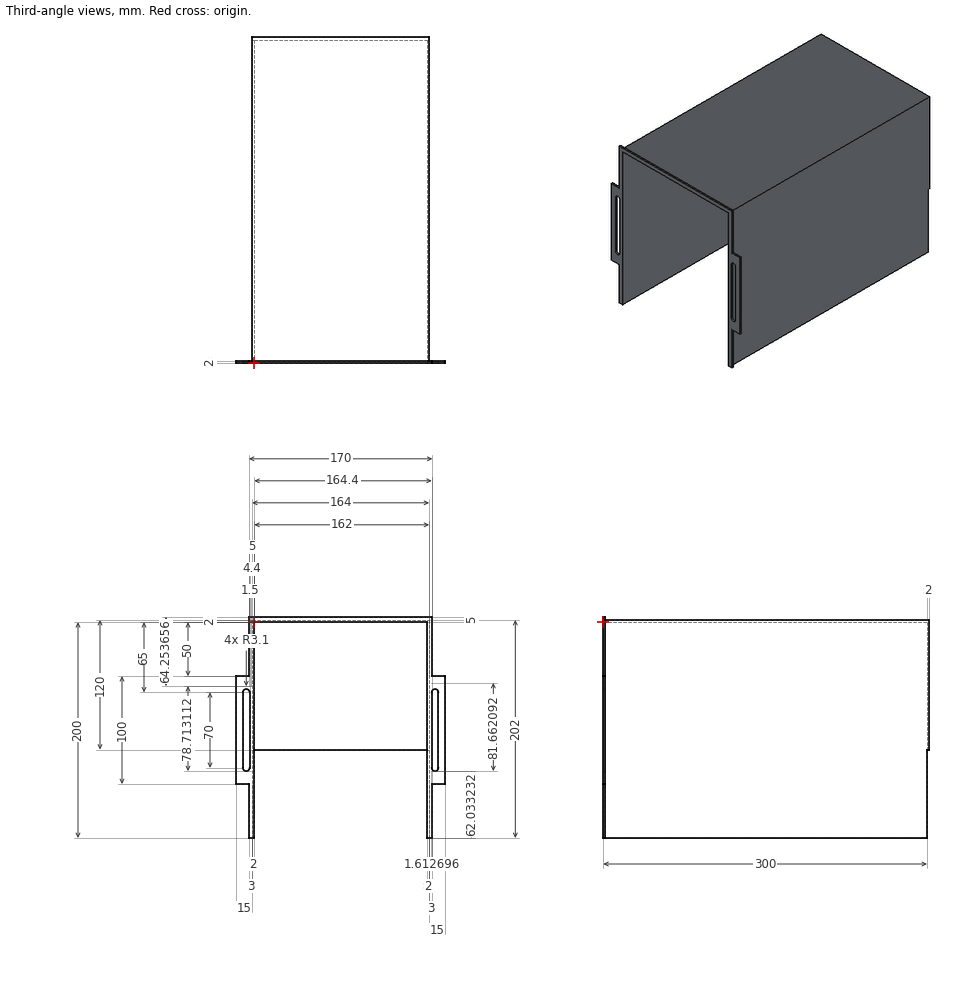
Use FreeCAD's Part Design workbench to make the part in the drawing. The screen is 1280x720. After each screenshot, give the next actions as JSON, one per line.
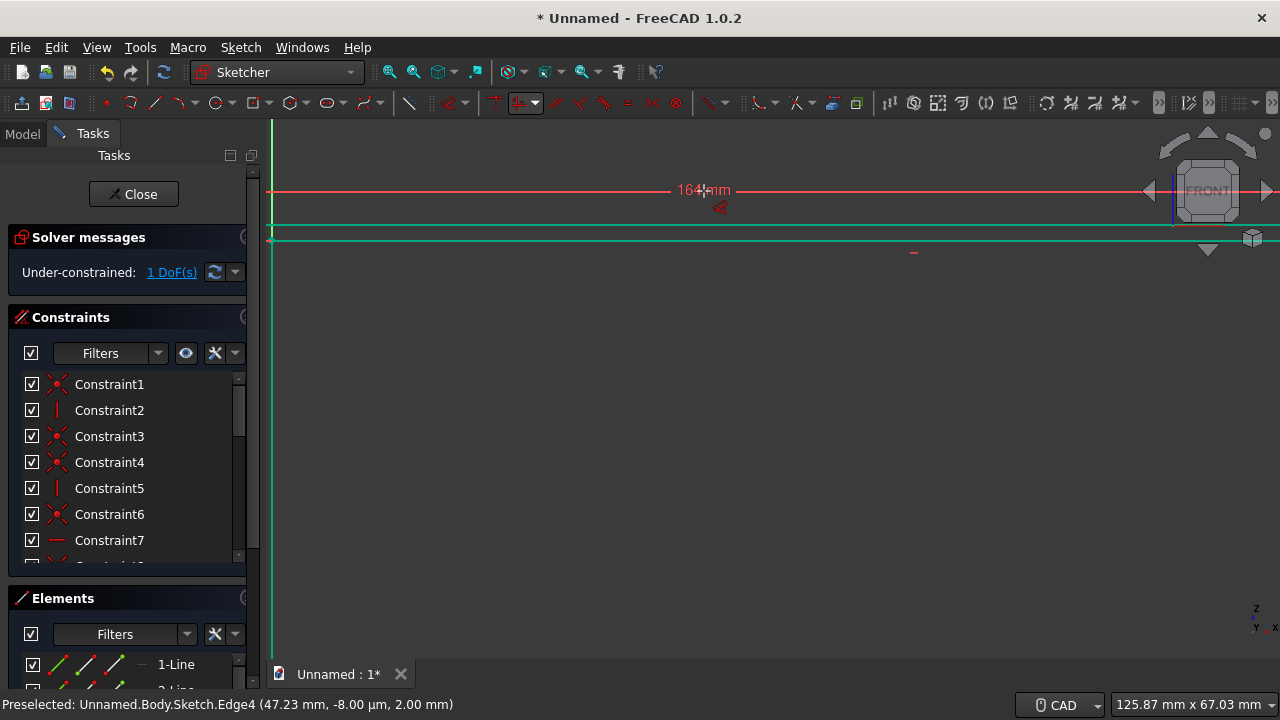
{"action": "scroll", "coordinate": [651, 225], "scroll_direction": "down", "scroll_amount": 8}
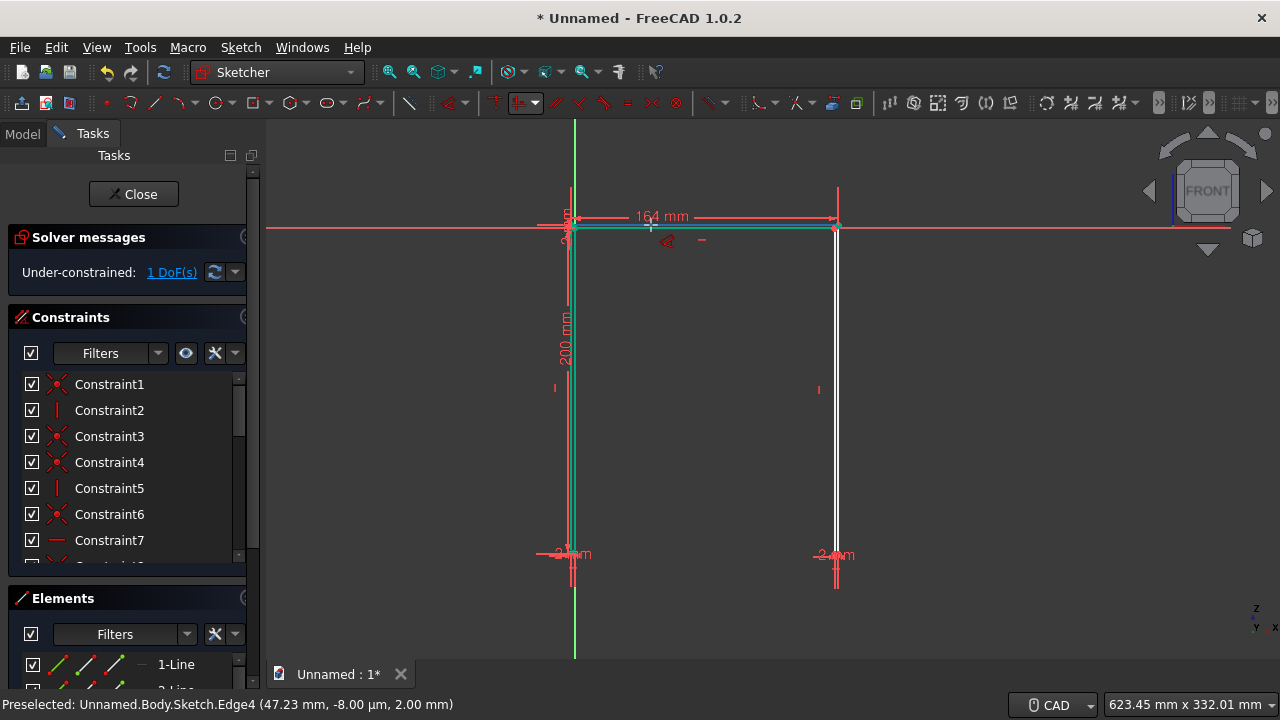
{"action": "scroll", "coordinate": [838, 324], "scroll_direction": "up", "scroll_amount": 8}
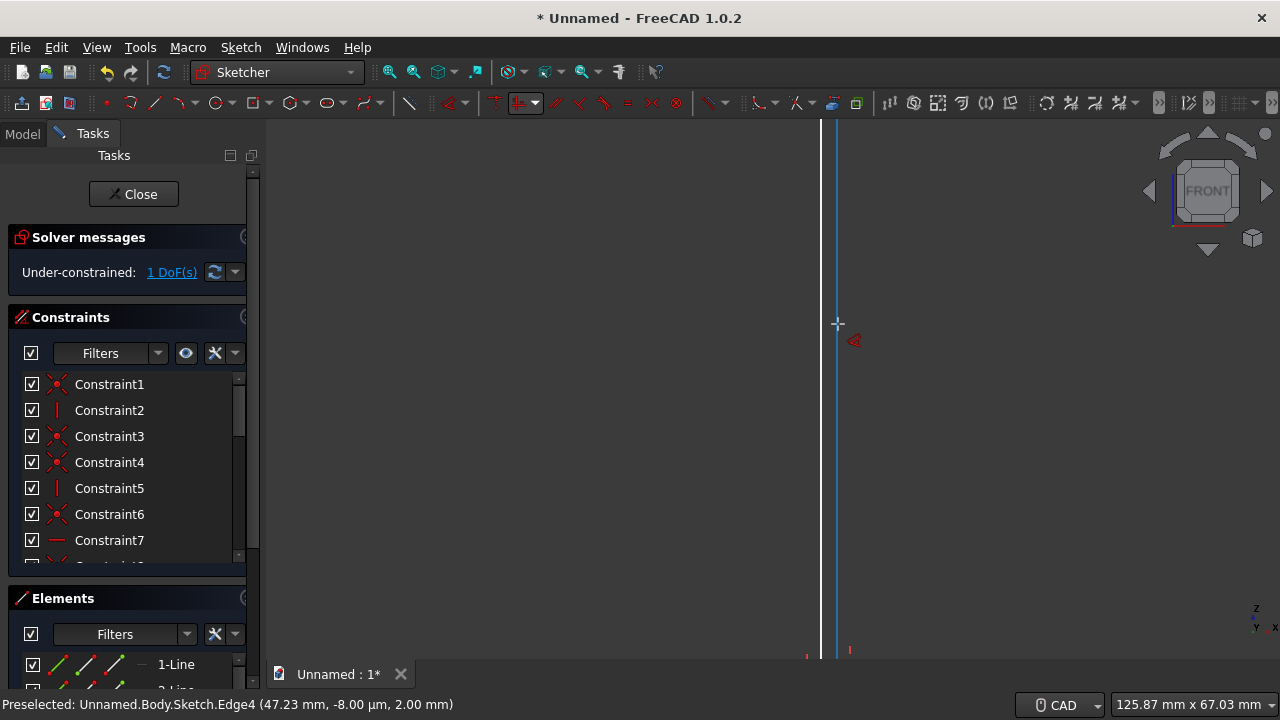
{"action": "left_click", "coordinate": [837, 323]}
{"action": "left_click", "coordinate": [871, 389]}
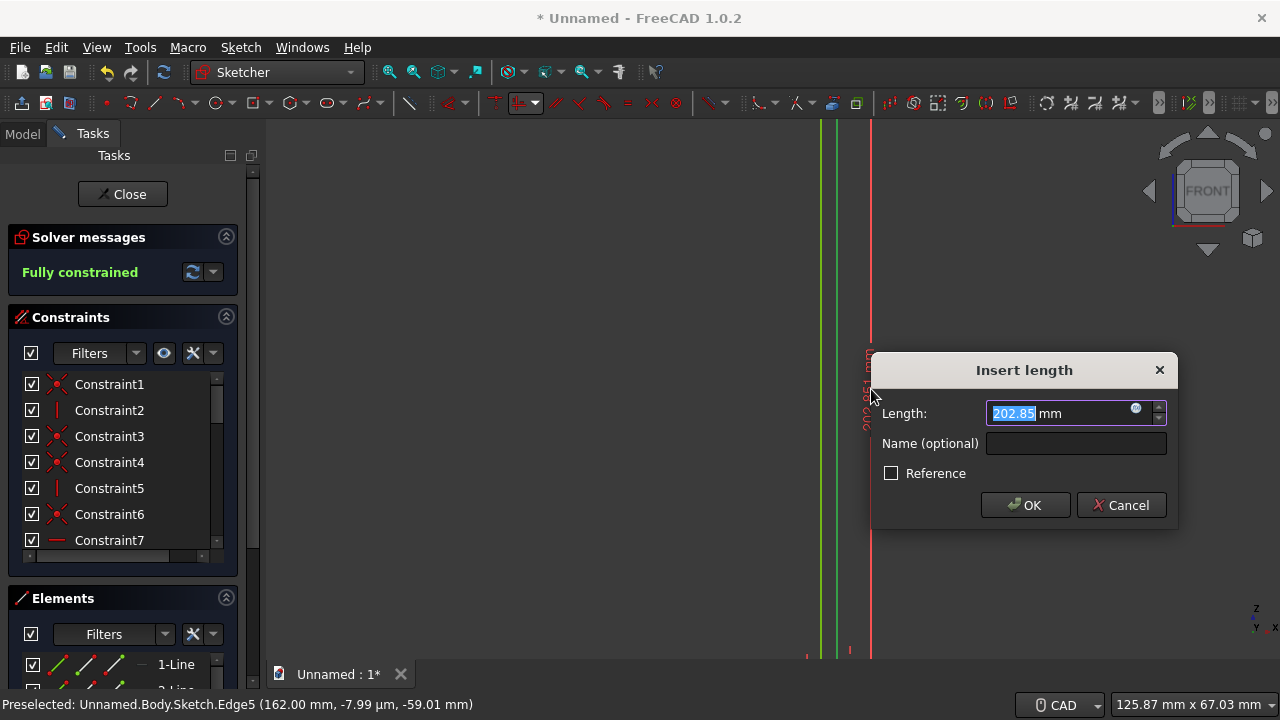
{"action": "type", "text": "202"}
{"action": "key", "text": "Return"}
{"action": "key", "text": "Escape"}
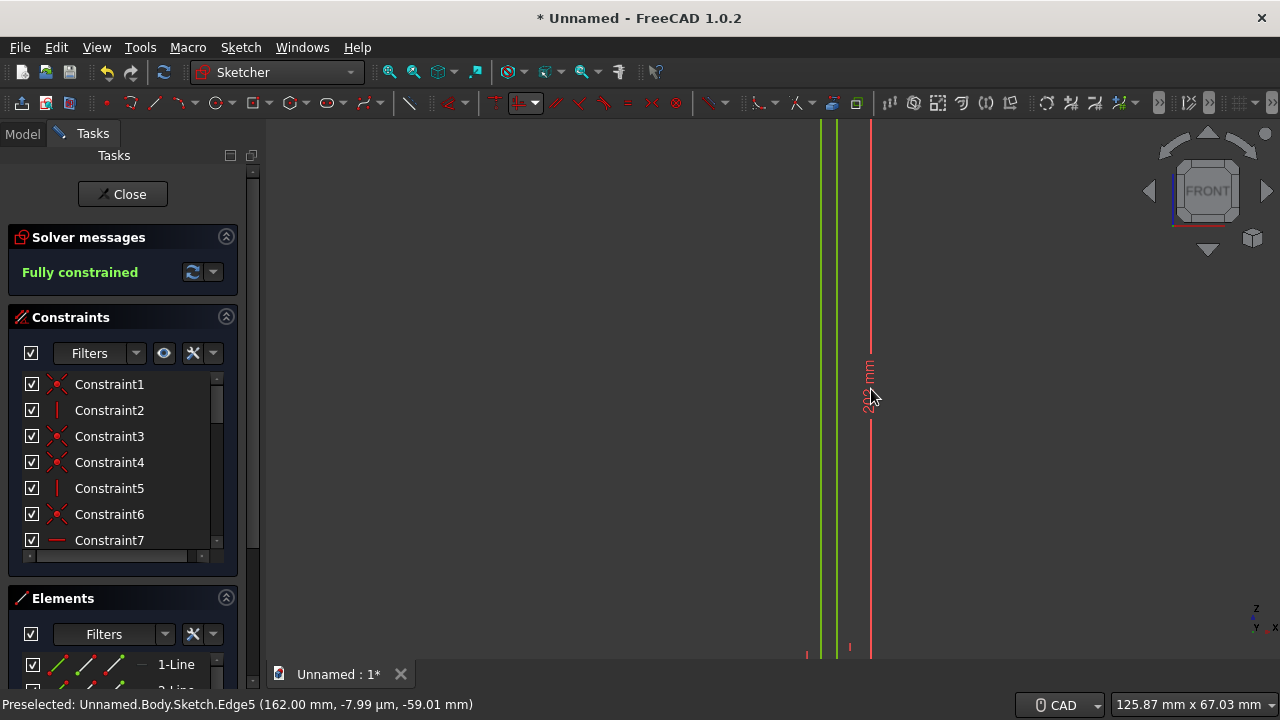
{"action": "left_click", "coordinate": [123, 194]}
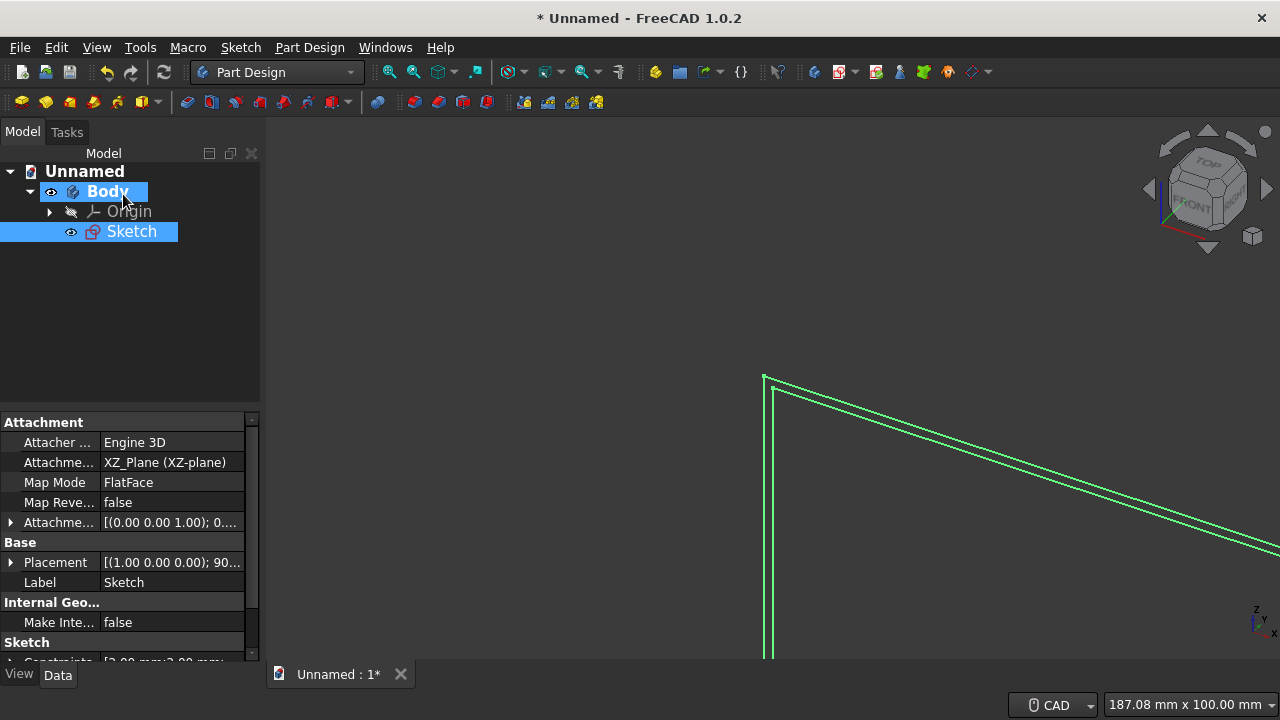
{"action": "left_click", "coordinate": [22, 102]}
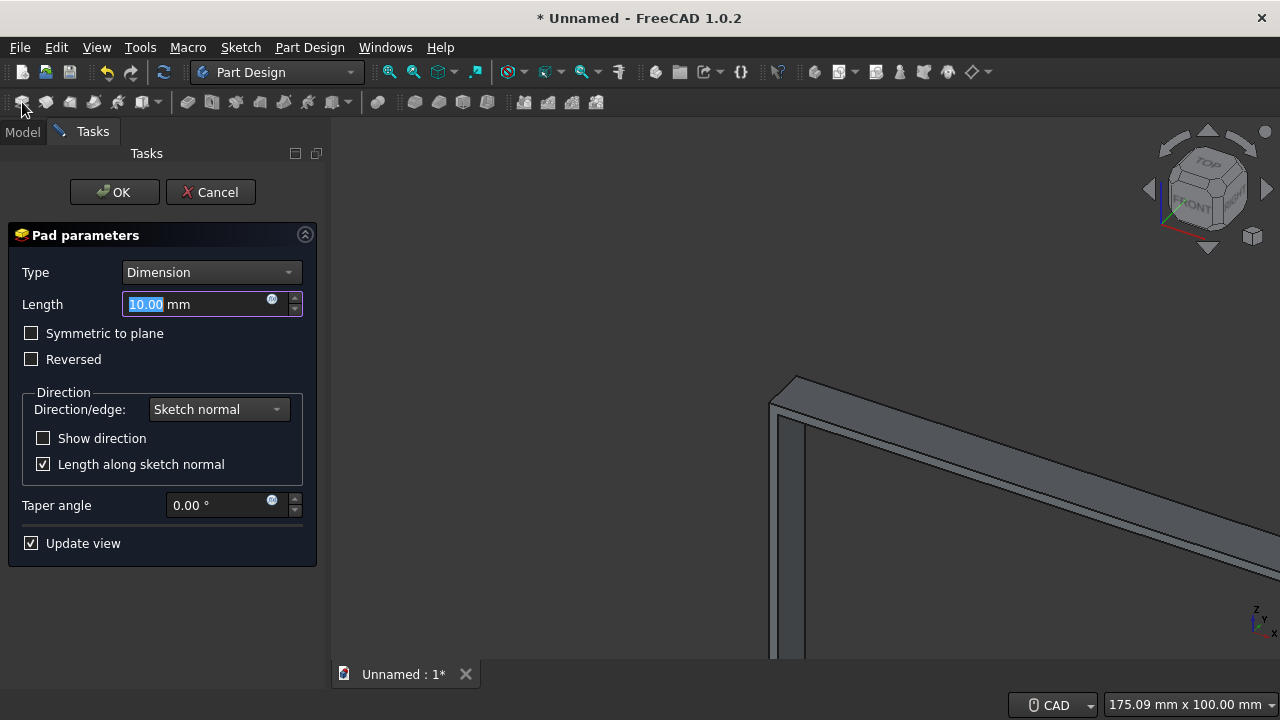
{"action": "type", "text": "300"}
{"action": "key", "text": "Tab"}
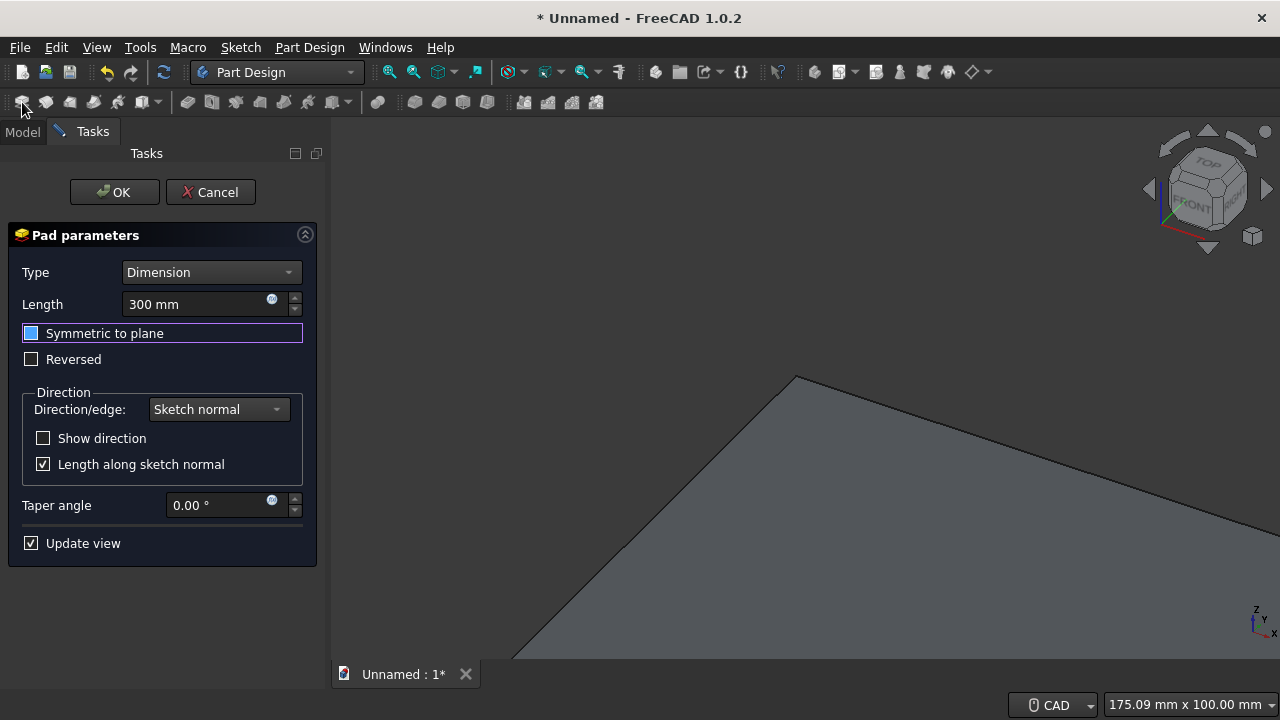
{"action": "left_click", "coordinate": [30, 359]}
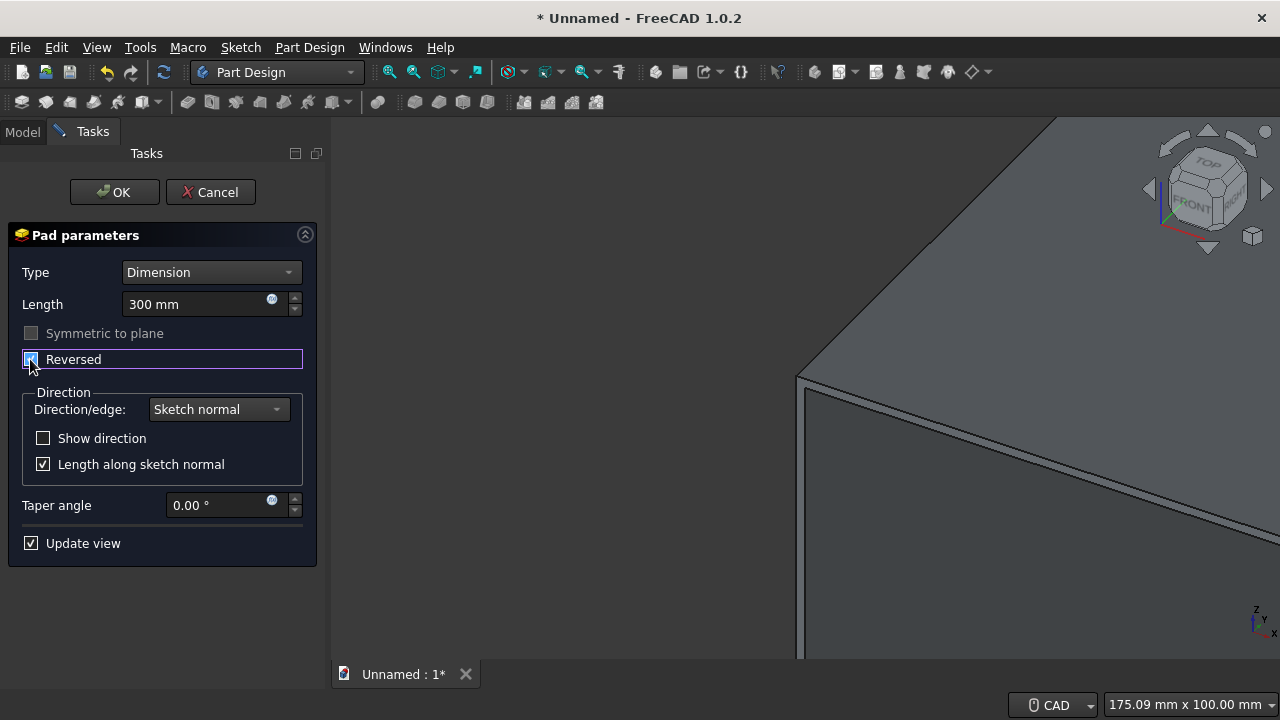
{"action": "left_click", "coordinate": [115, 192]}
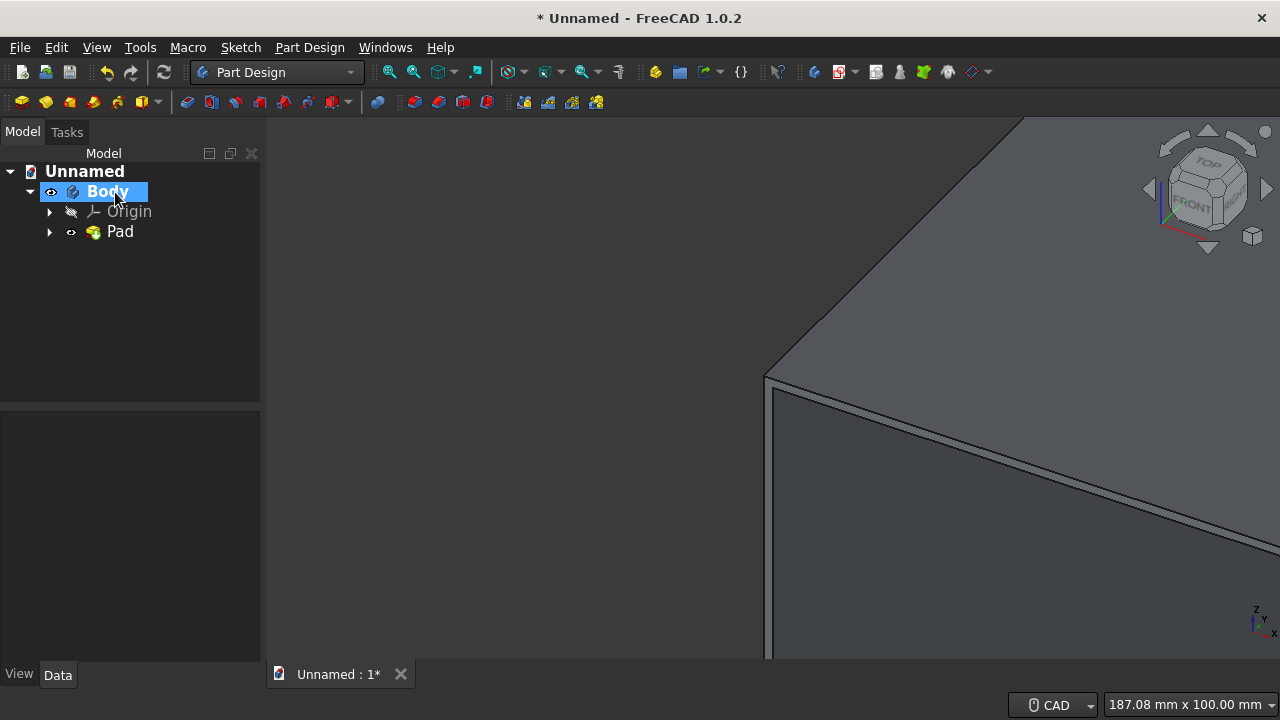
{"action": "left_click", "coordinate": [390, 72]}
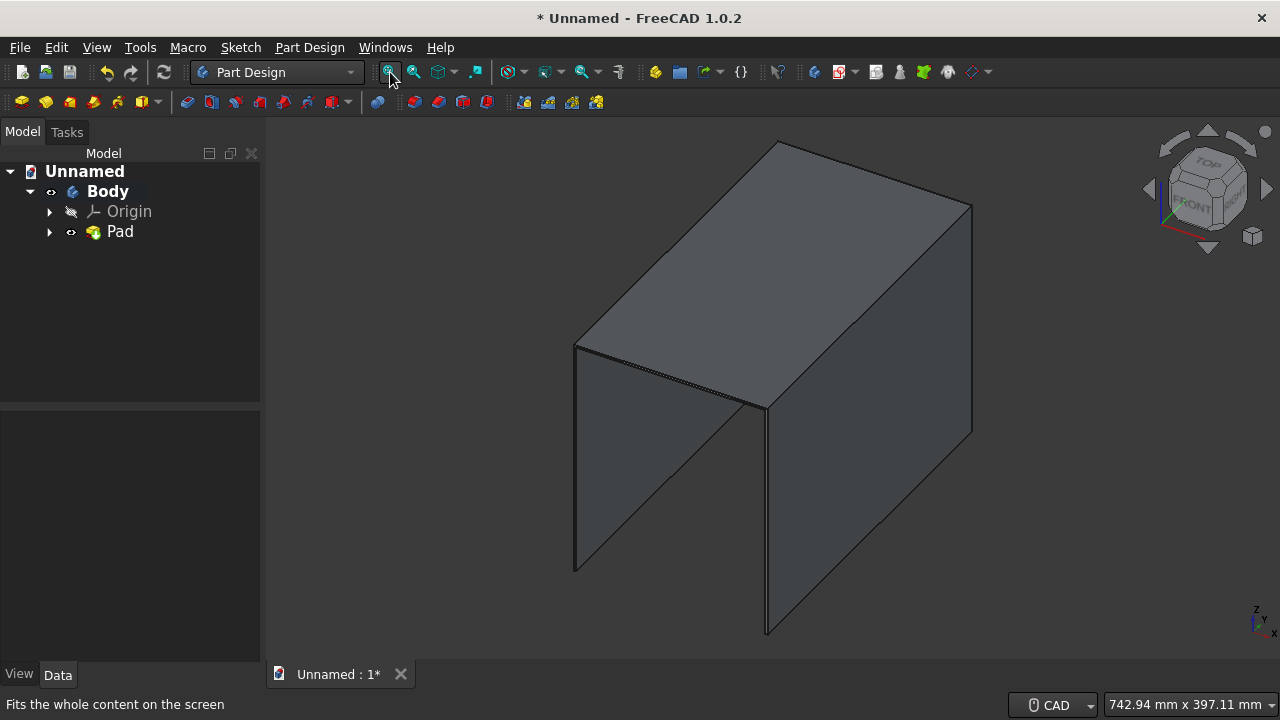
{"action": "scroll", "coordinate": [766, 559], "scroll_direction": "up", "scroll_amount": 13}